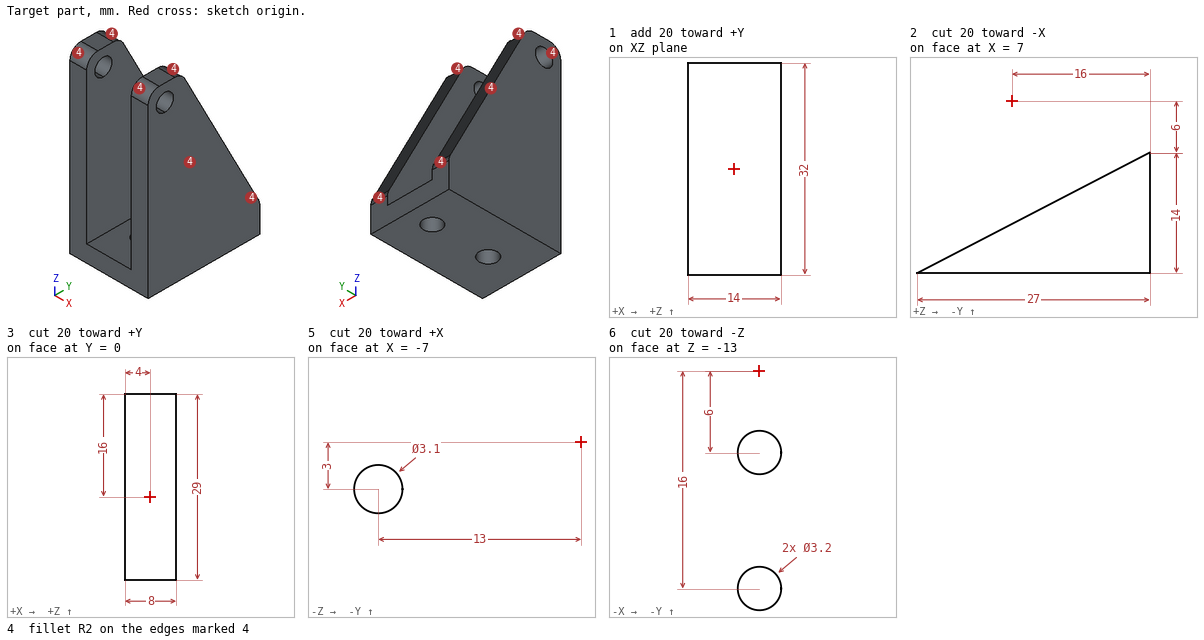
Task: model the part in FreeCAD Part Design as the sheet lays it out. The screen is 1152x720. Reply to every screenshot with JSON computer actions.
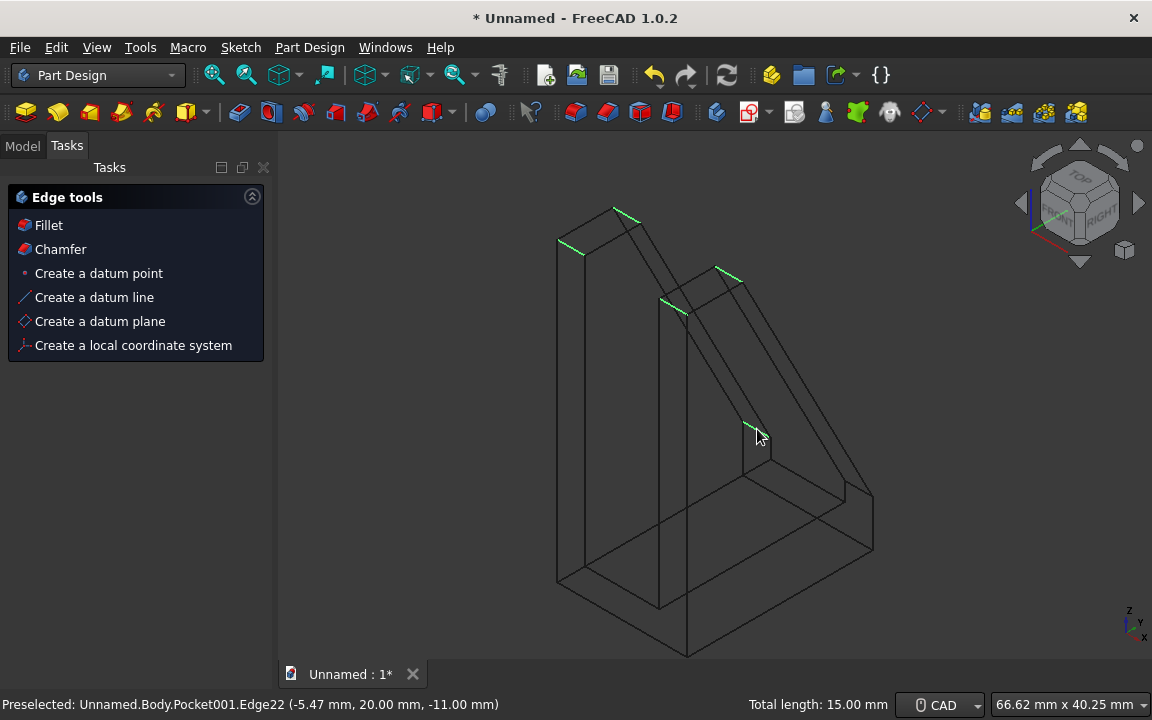
{"action": "left_click", "coordinate": [859, 488], "text": "ctrl"}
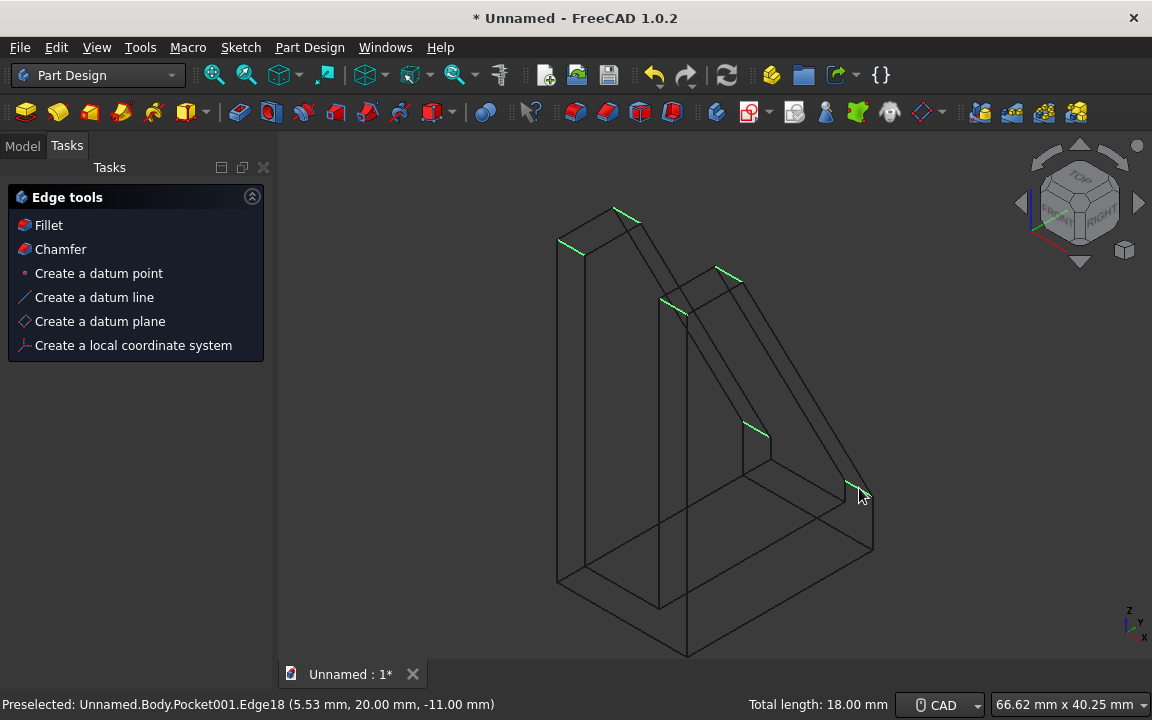
{"action": "key", "text": "v 1"}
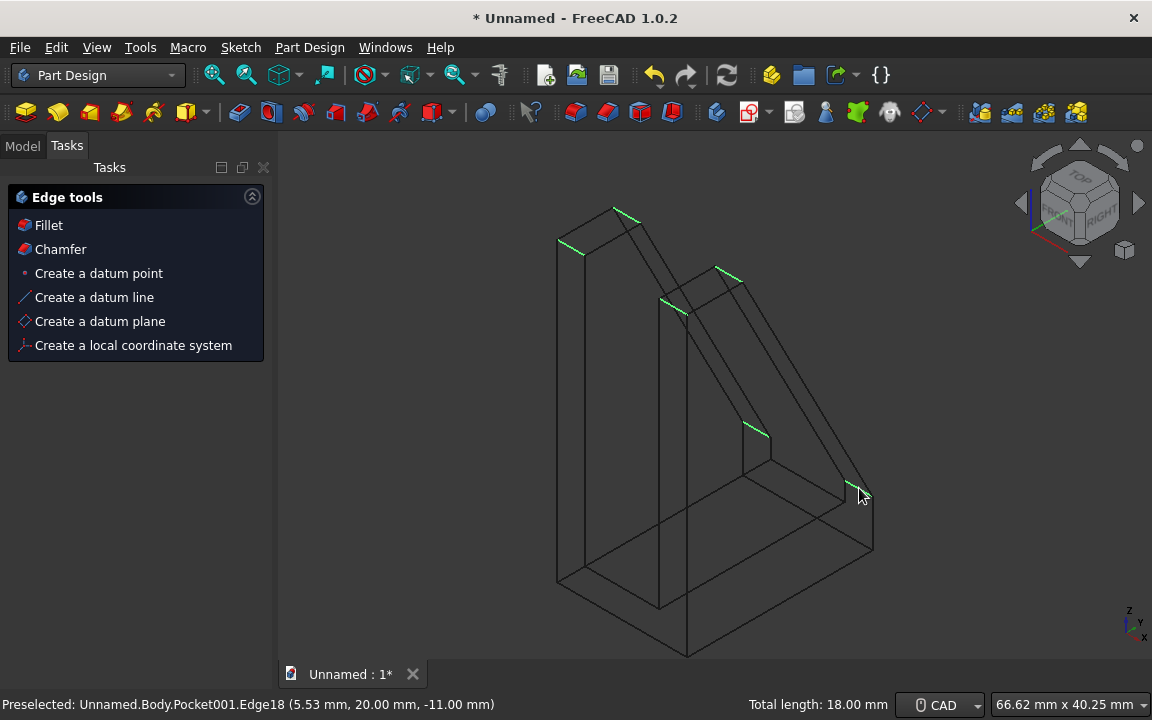
{"action": "left_click", "coordinate": [576, 112]}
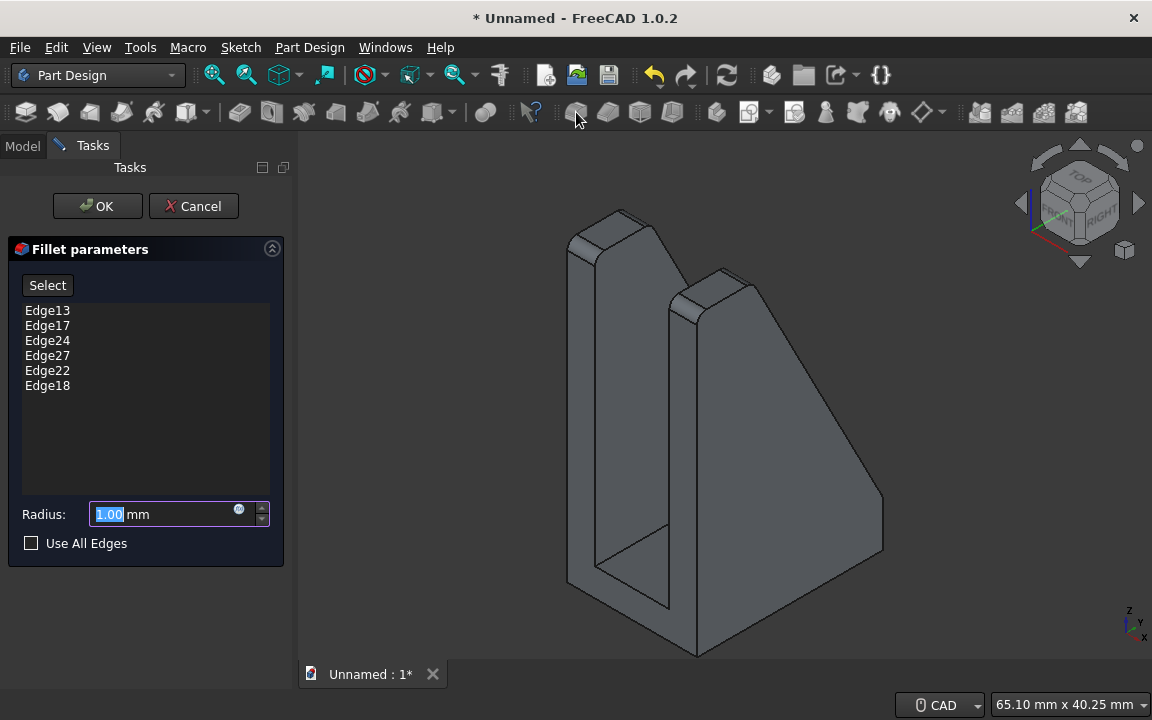
{"action": "type", "text": "2"}
{"action": "key", "text": "Tab"}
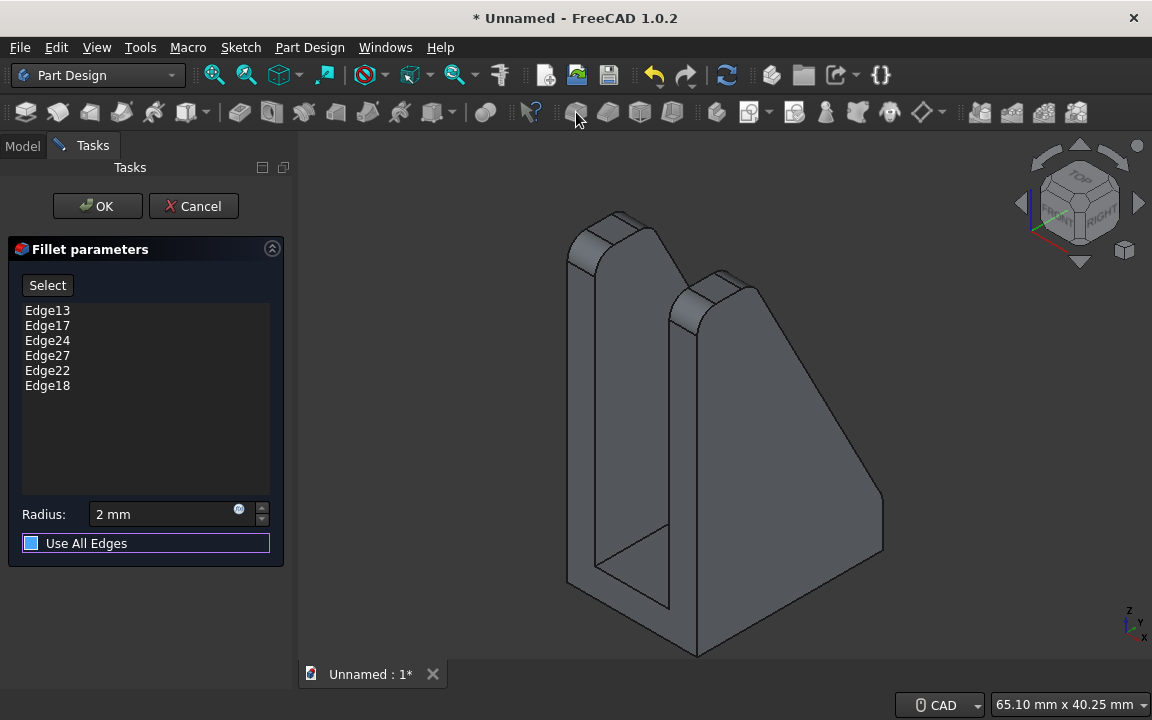
{"action": "left_click", "coordinate": [98, 206]}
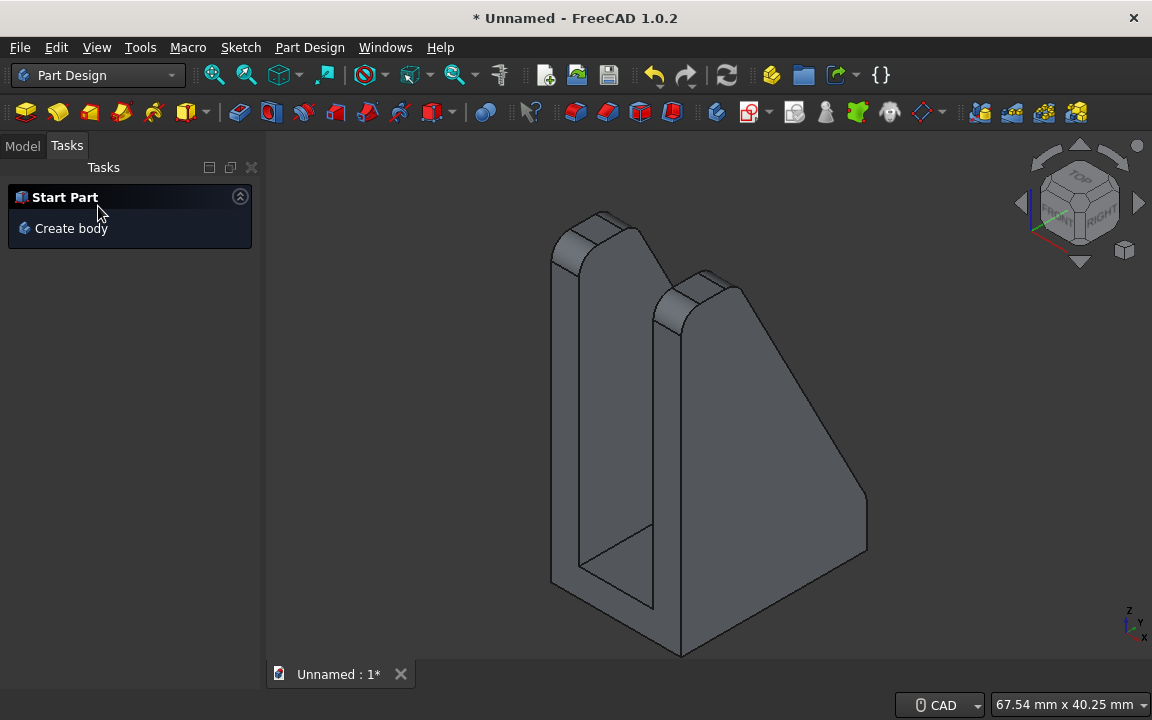
{"action": "key", "text": "6"}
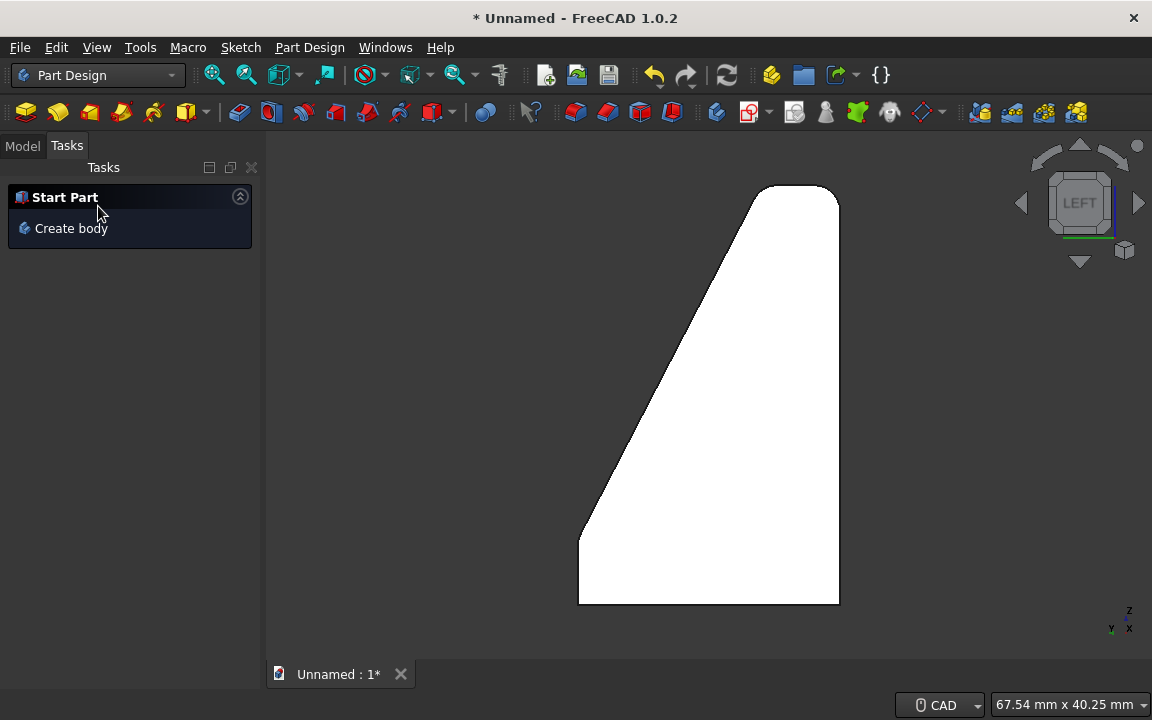
{"action": "left_click", "coordinate": [746, 454]}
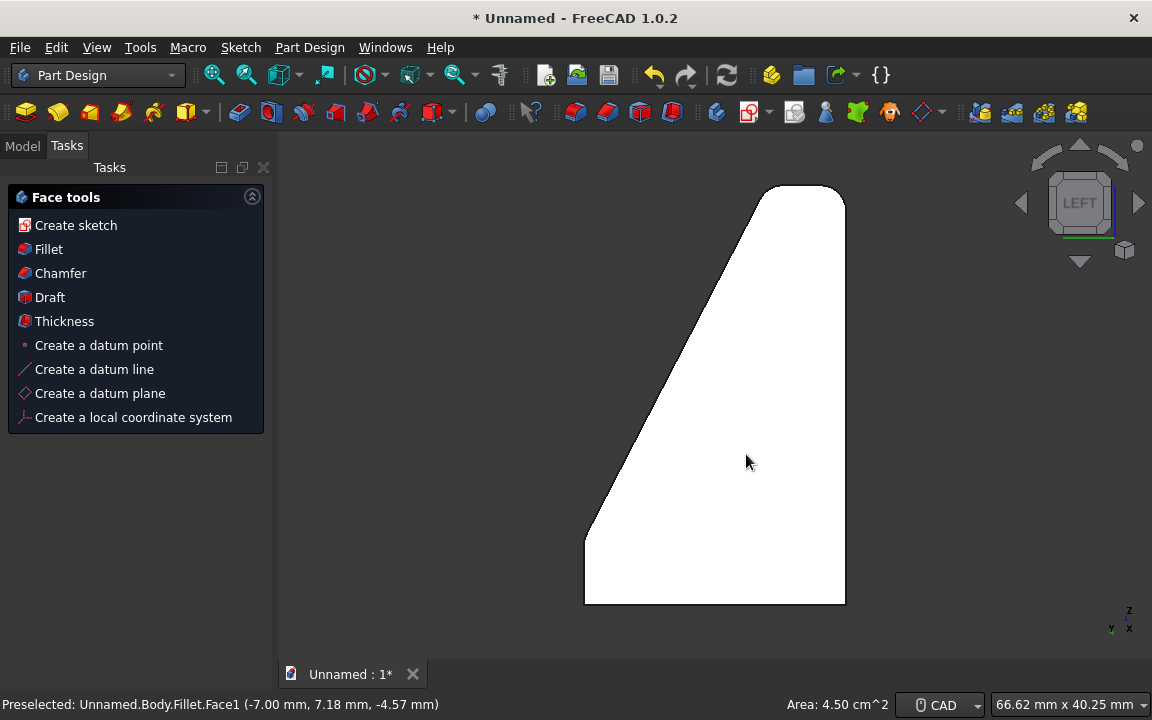
{"action": "left_click", "coordinate": [750, 112]}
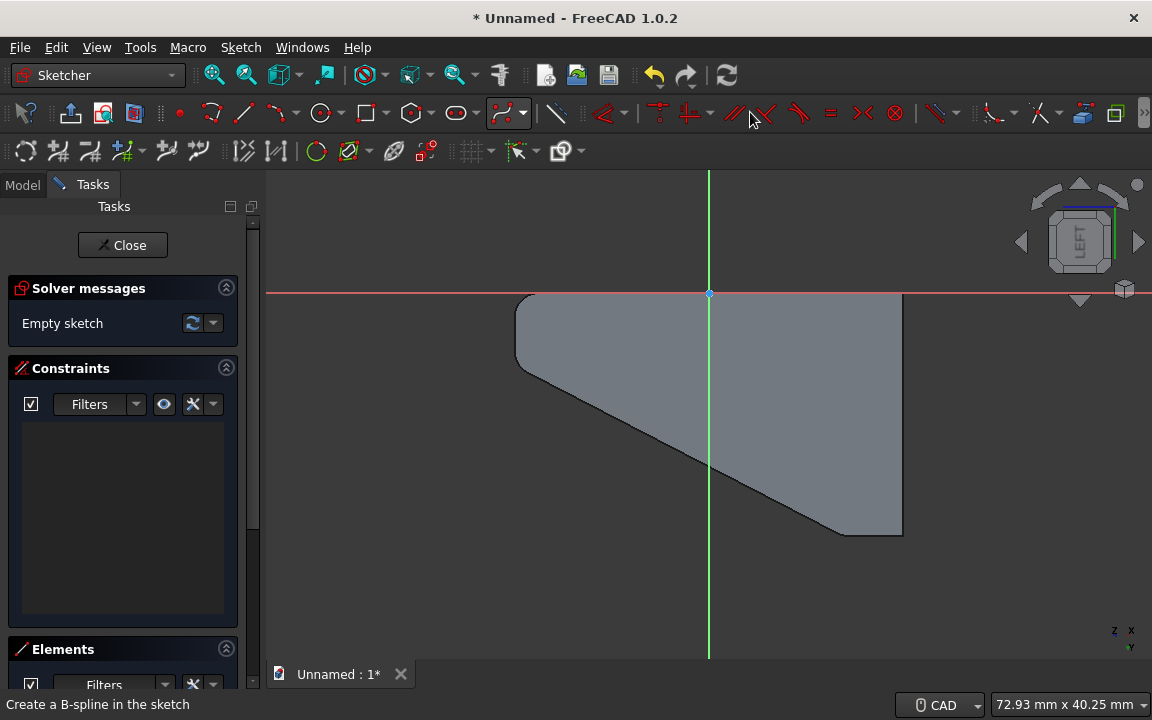
{"action": "scroll", "coordinate": [537, 316], "scroll_direction": "up", "scroll_amount": 10}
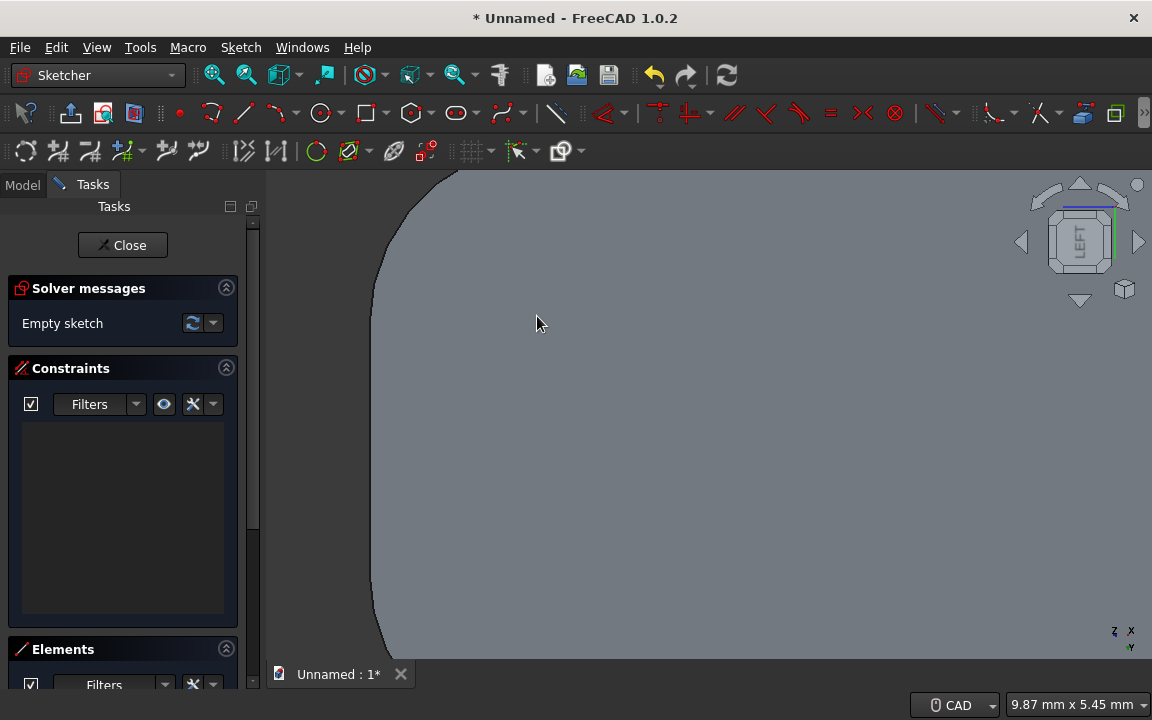
{"action": "left_click", "coordinate": [322, 114]}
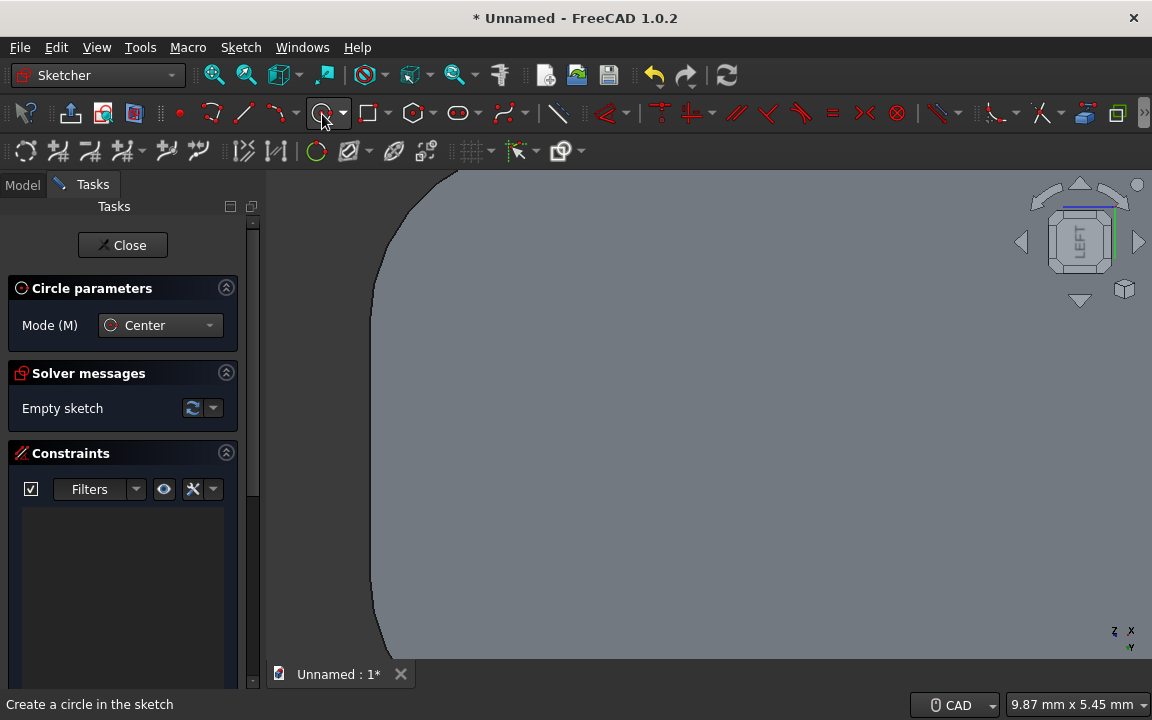
{"action": "left_click", "coordinate": [639, 414]}
{"action": "mouse_move", "coordinate": [737, 315]}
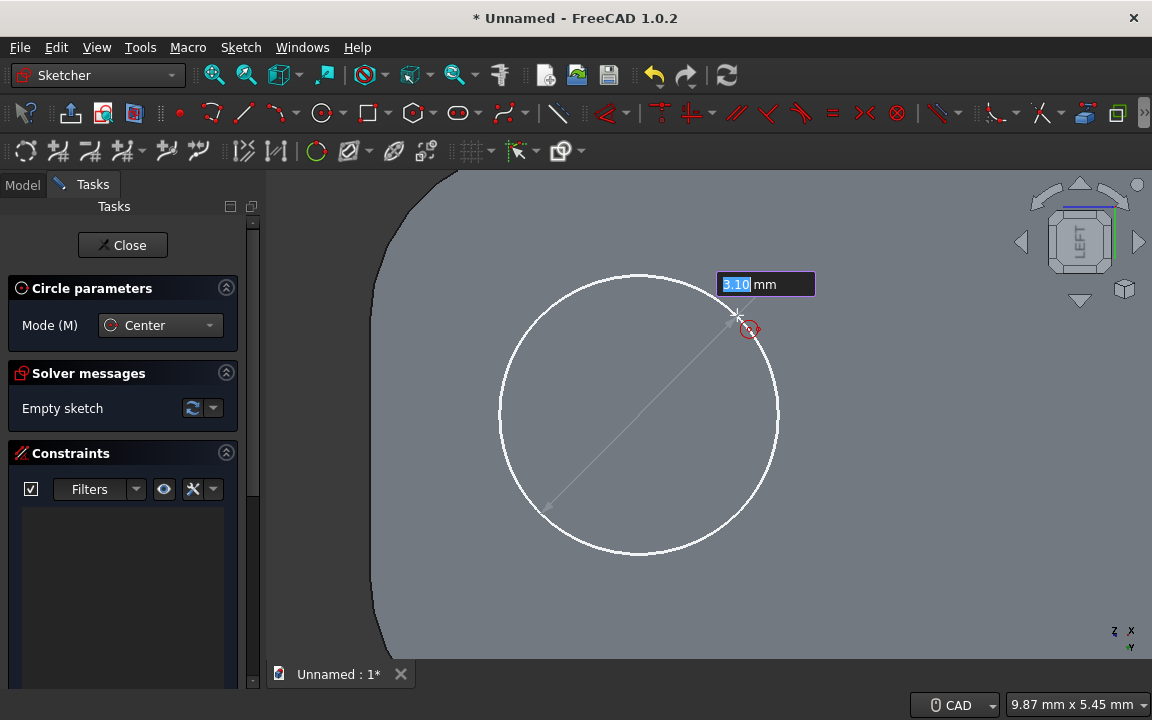
{"action": "type", "text": "3.1"}
{"action": "key", "text": "Return"}
{"action": "key", "text": "Escape"}